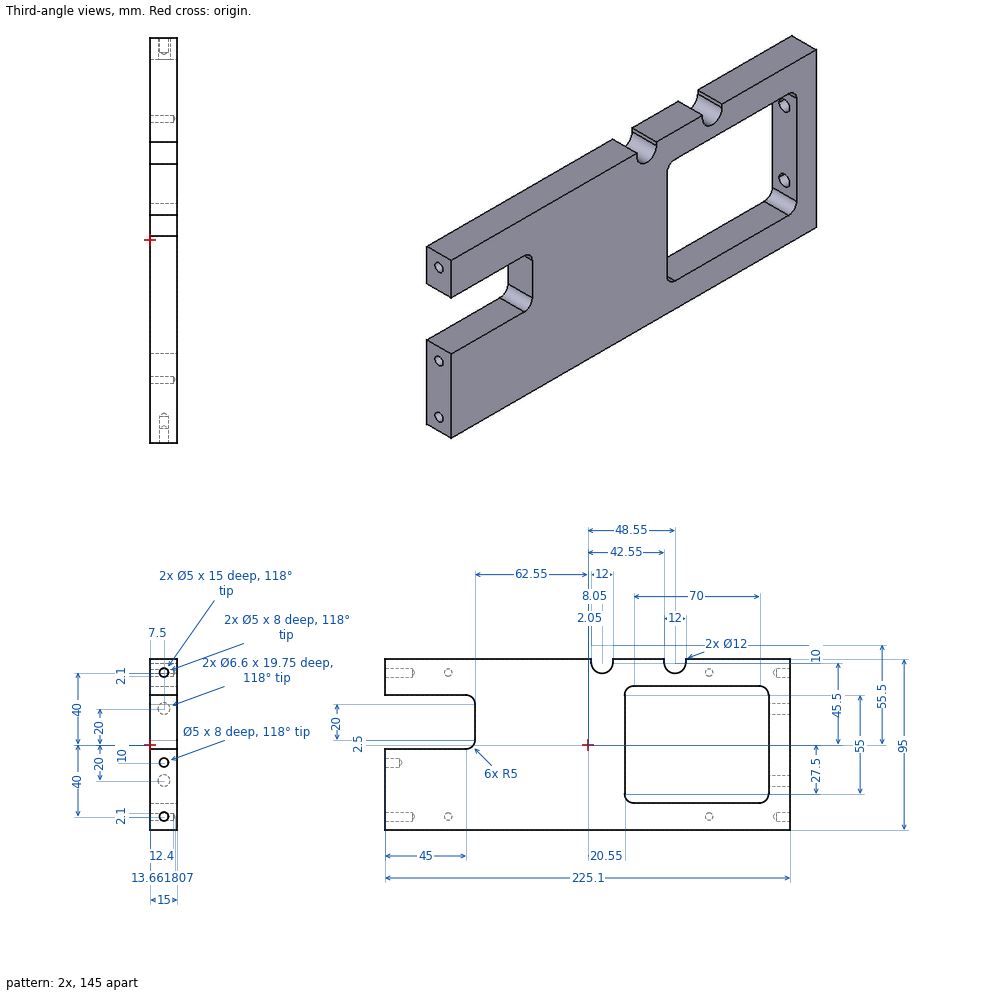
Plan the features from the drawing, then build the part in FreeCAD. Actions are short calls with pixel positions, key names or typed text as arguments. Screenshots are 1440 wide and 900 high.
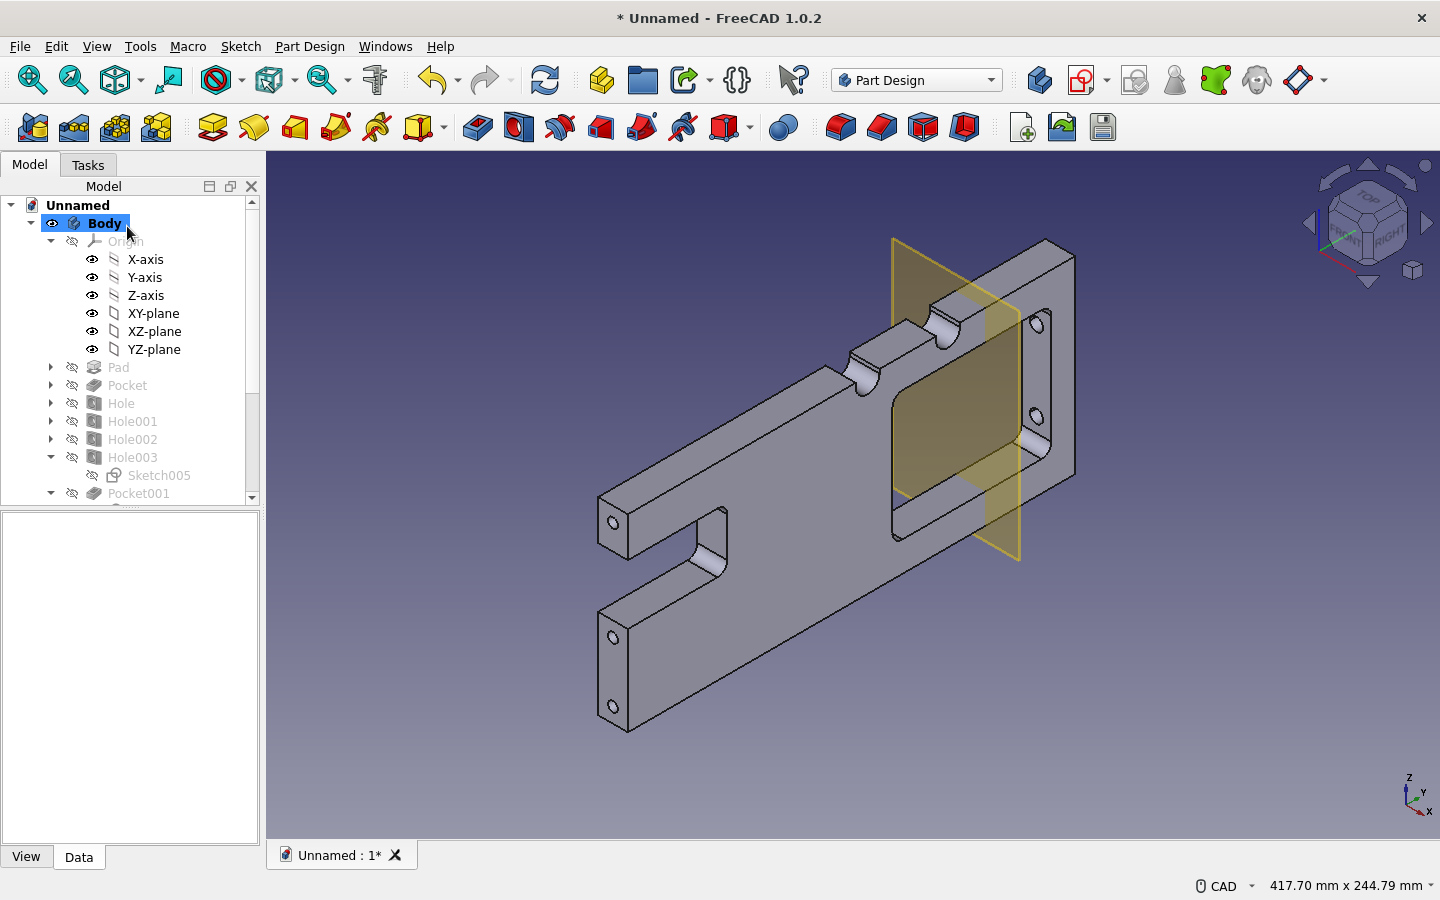
scroll(101, 345, down, 3)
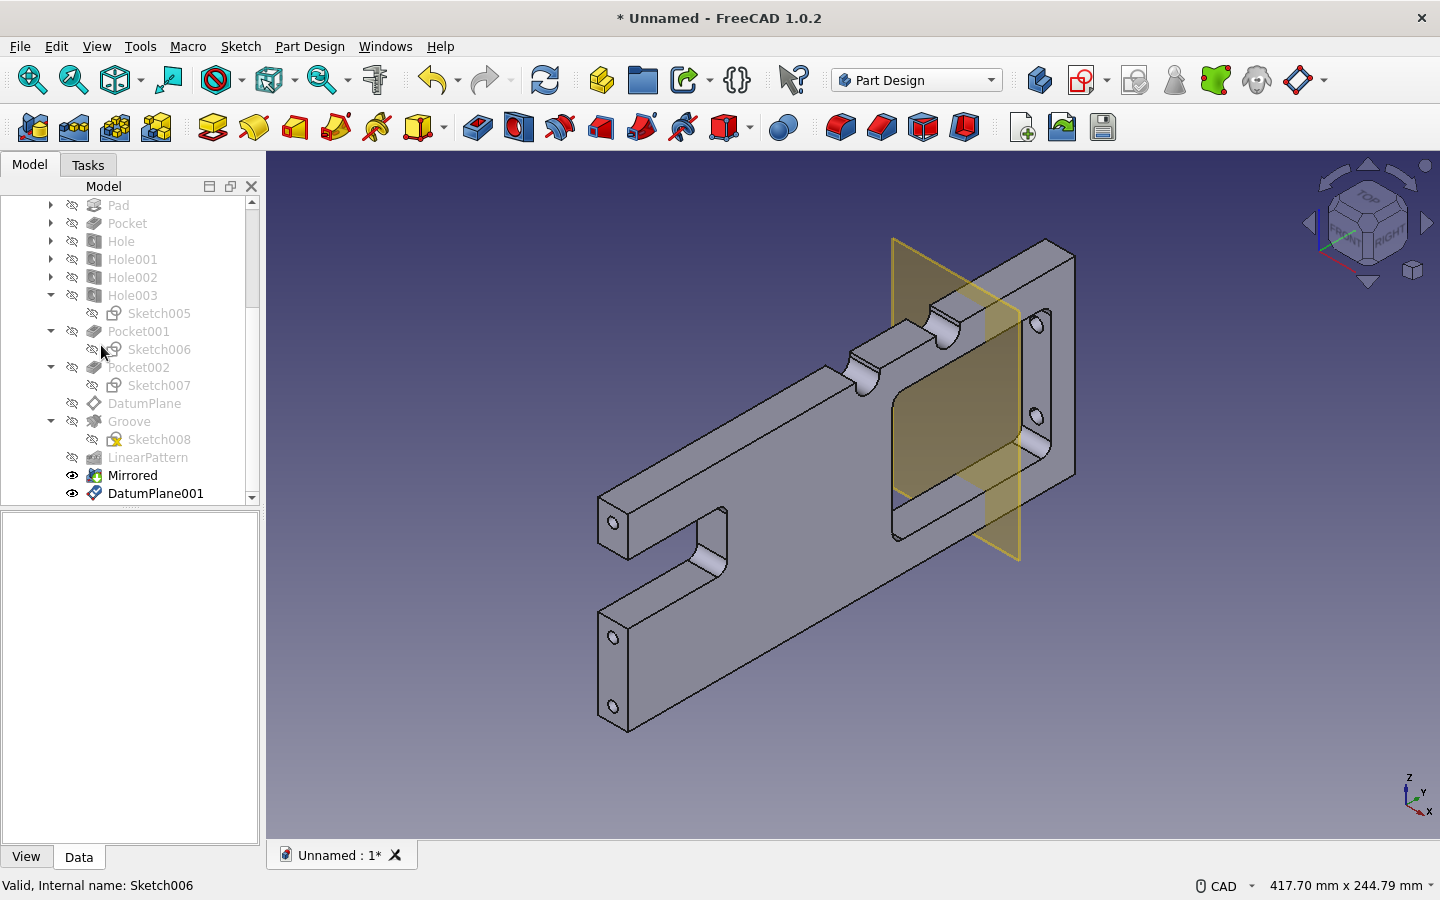
click(117, 493)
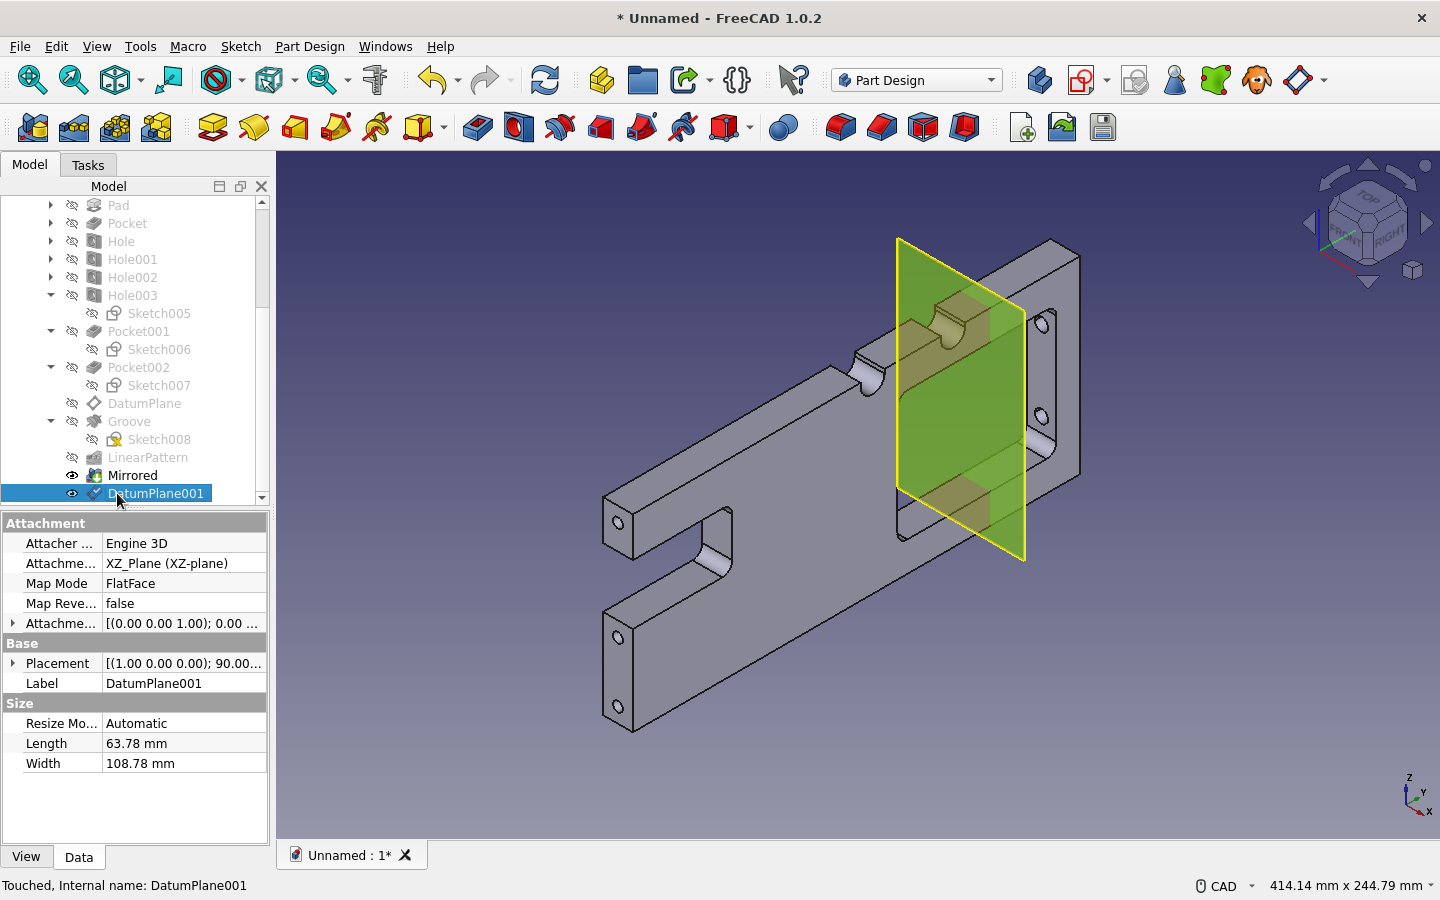
click(1080, 80)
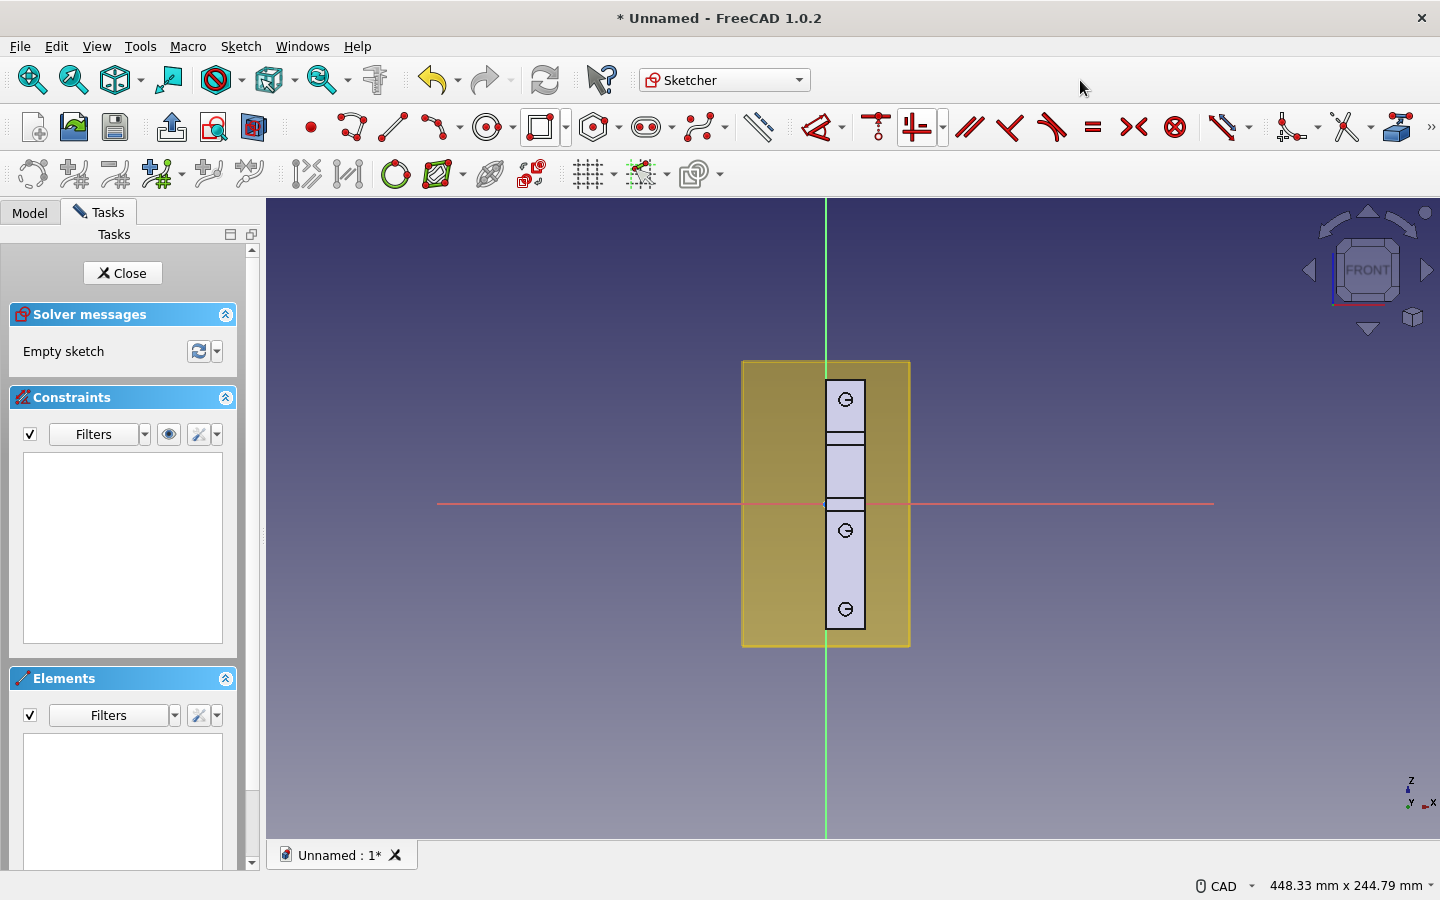
click(254, 128)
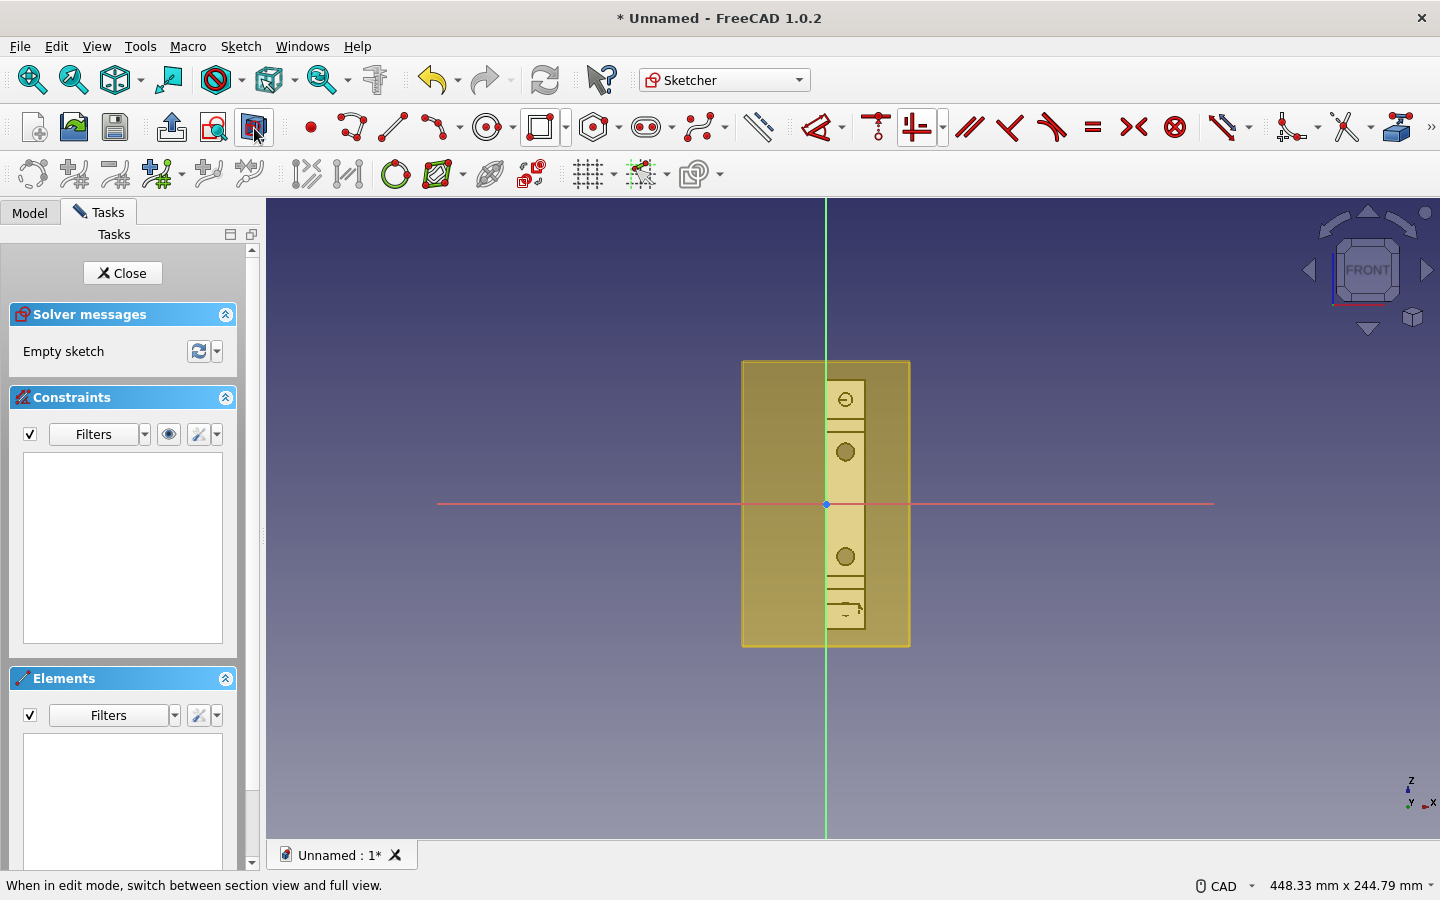
scroll(854, 430, up, 7)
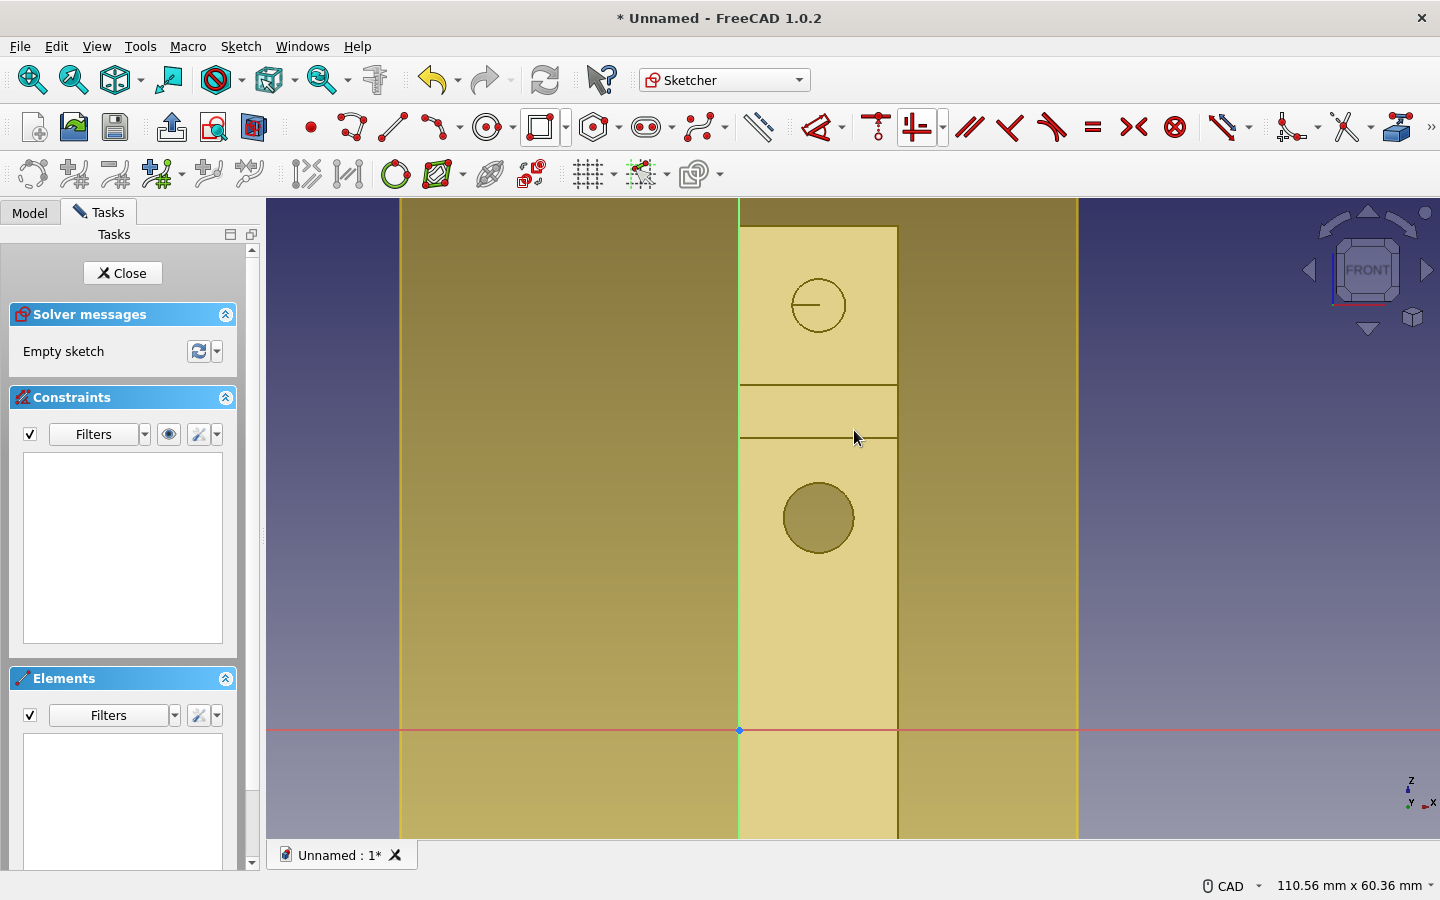
click(352, 128)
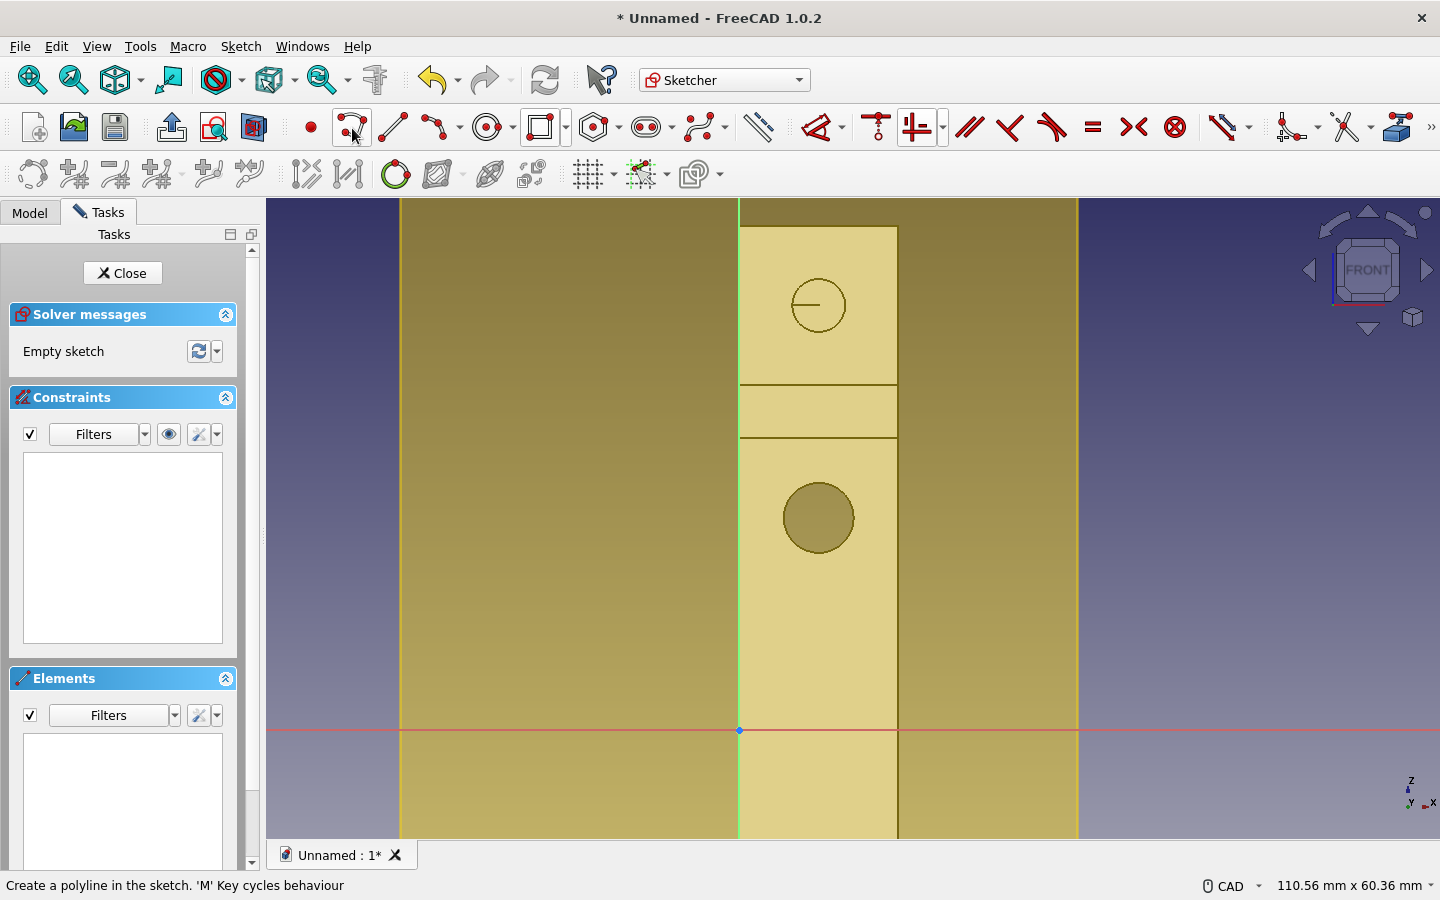
click(739, 328)
click(748, 305)
click(884, 305)
click(871, 328)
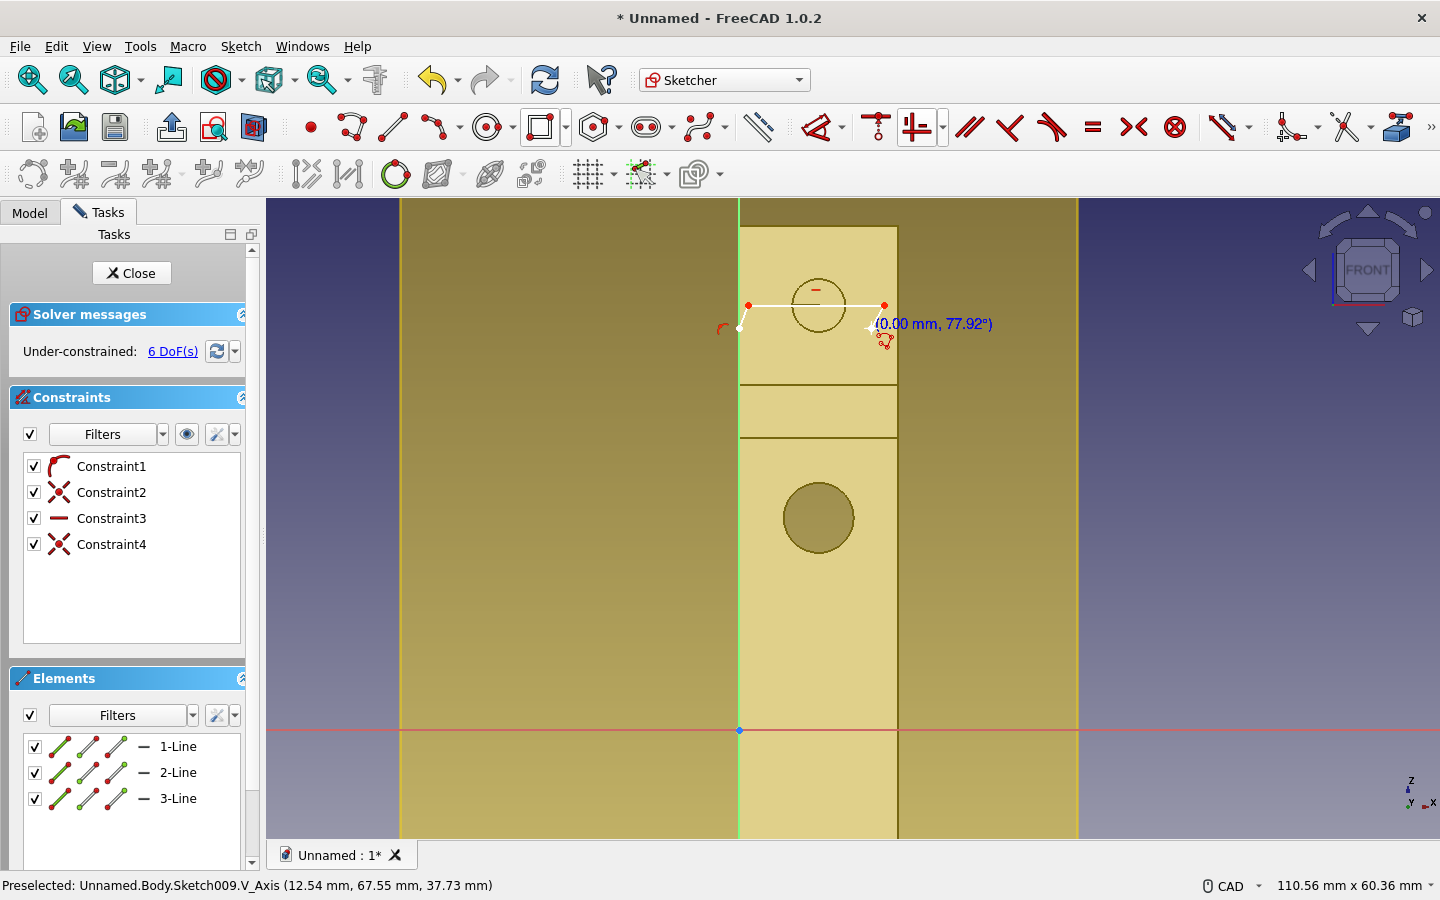
scroll(739, 328, up, 2)